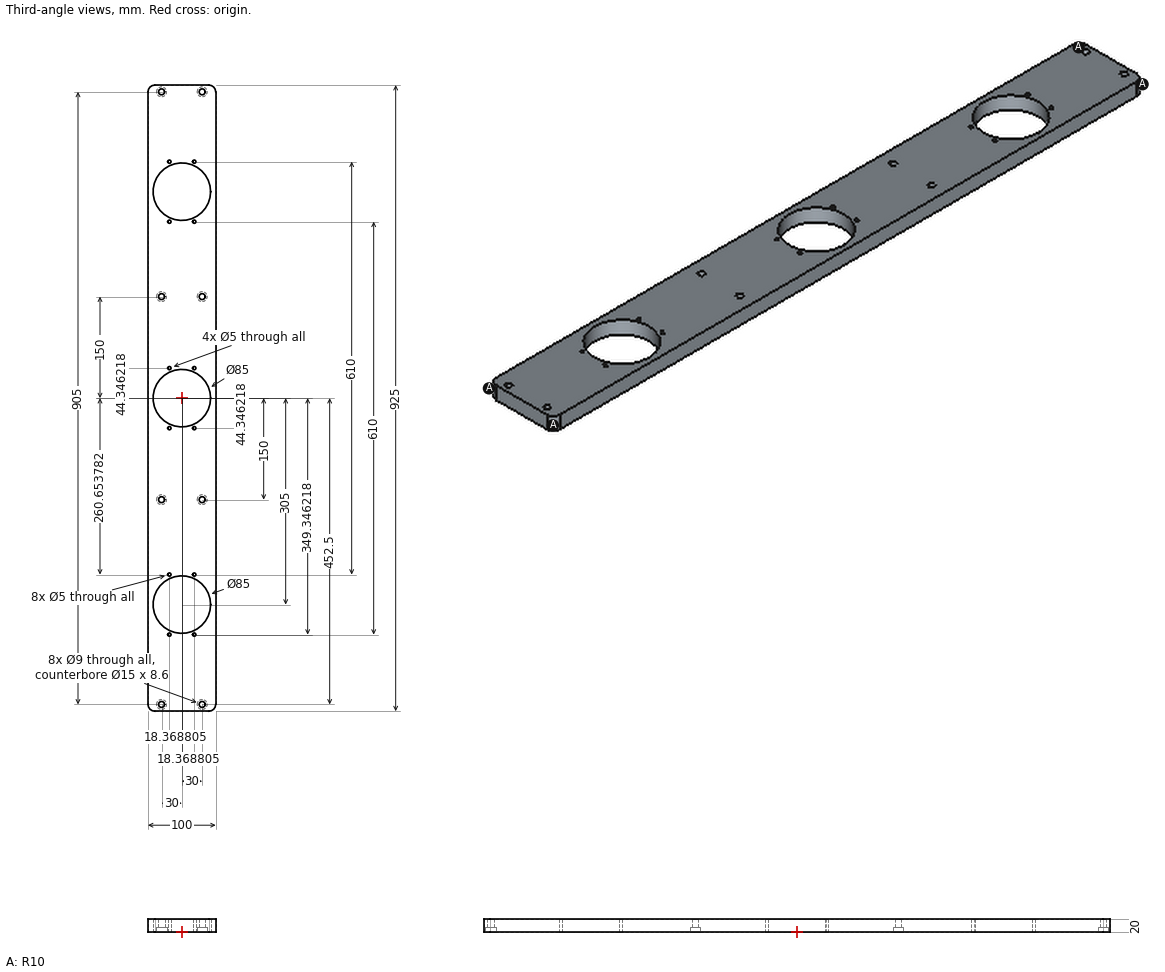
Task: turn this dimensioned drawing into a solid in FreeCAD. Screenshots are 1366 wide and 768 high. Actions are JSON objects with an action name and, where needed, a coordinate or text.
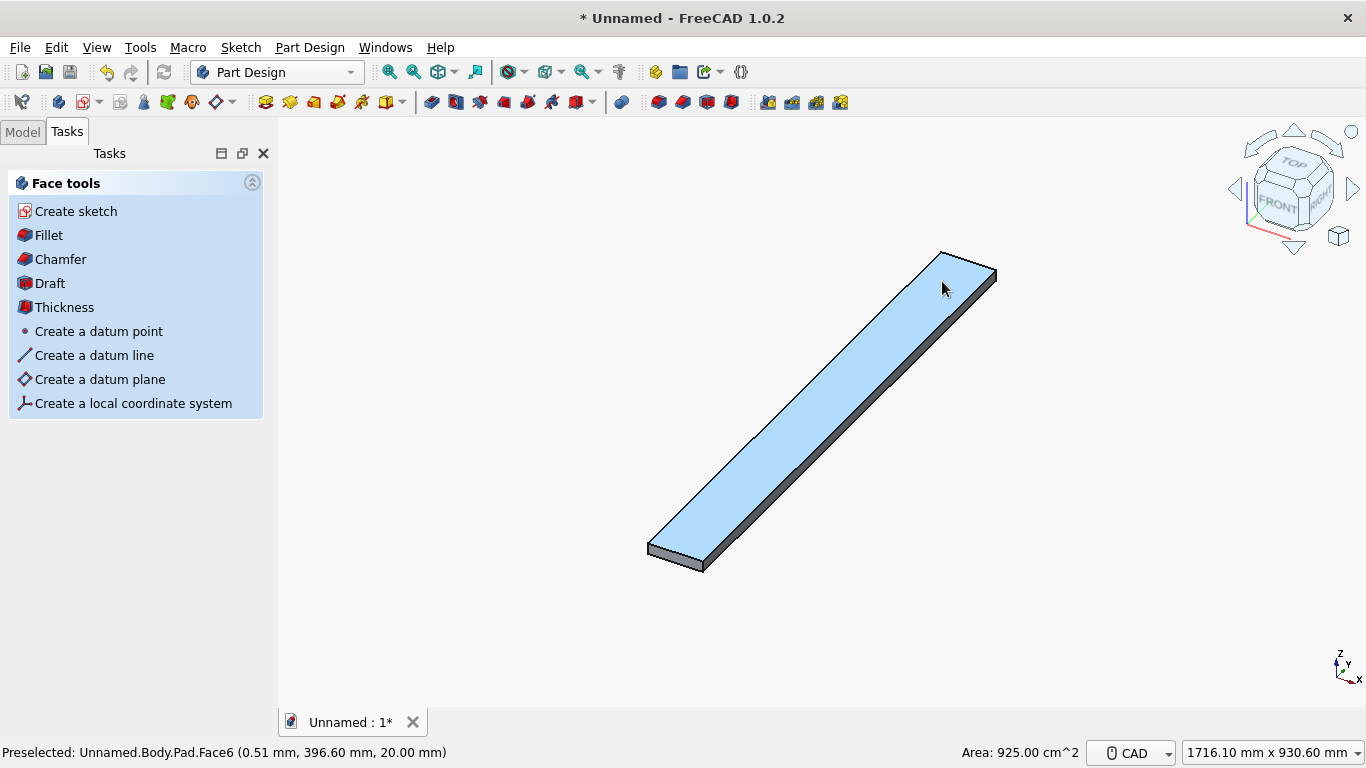
{"action": "left_click", "coordinate": [84, 102]}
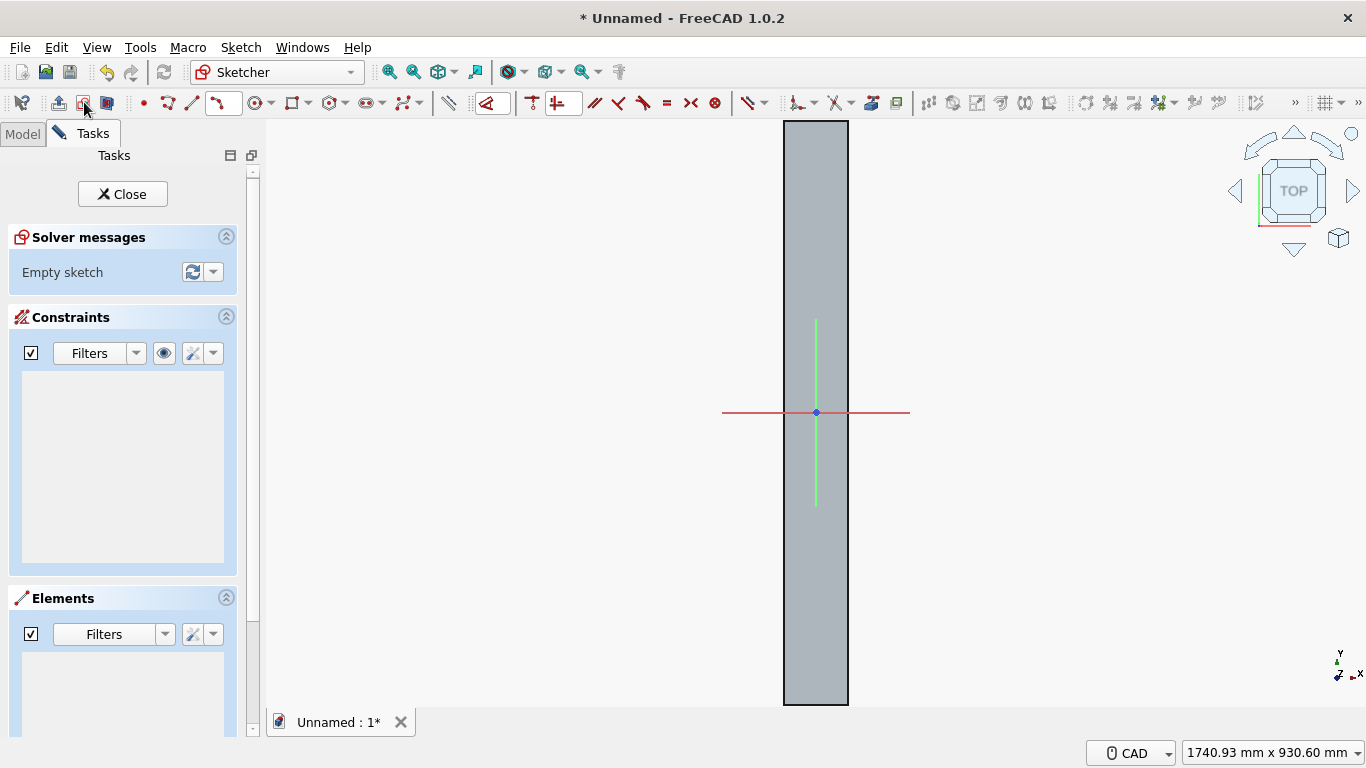
{"action": "left_click", "coordinate": [256, 104]}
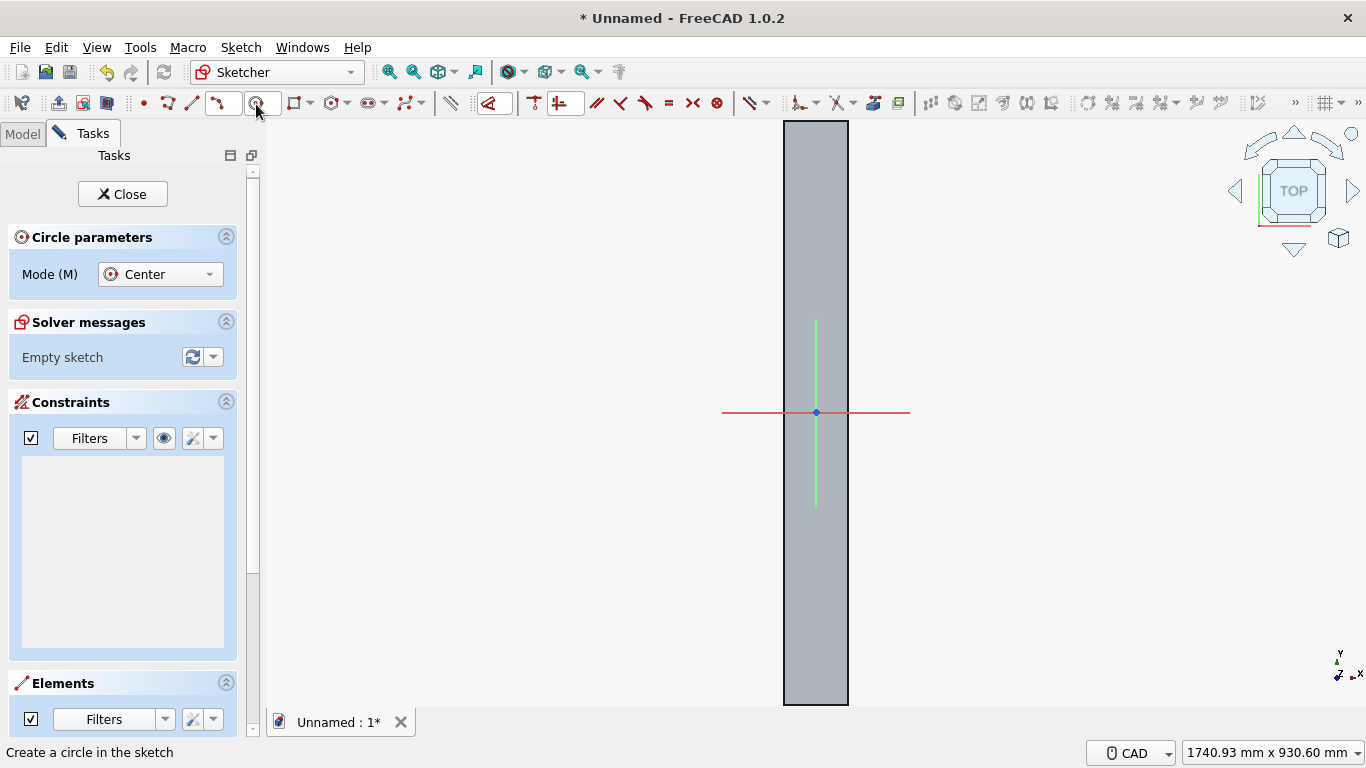
{"action": "scroll", "coordinate": [804, 578], "scroll_direction": "up", "scroll_amount": 14}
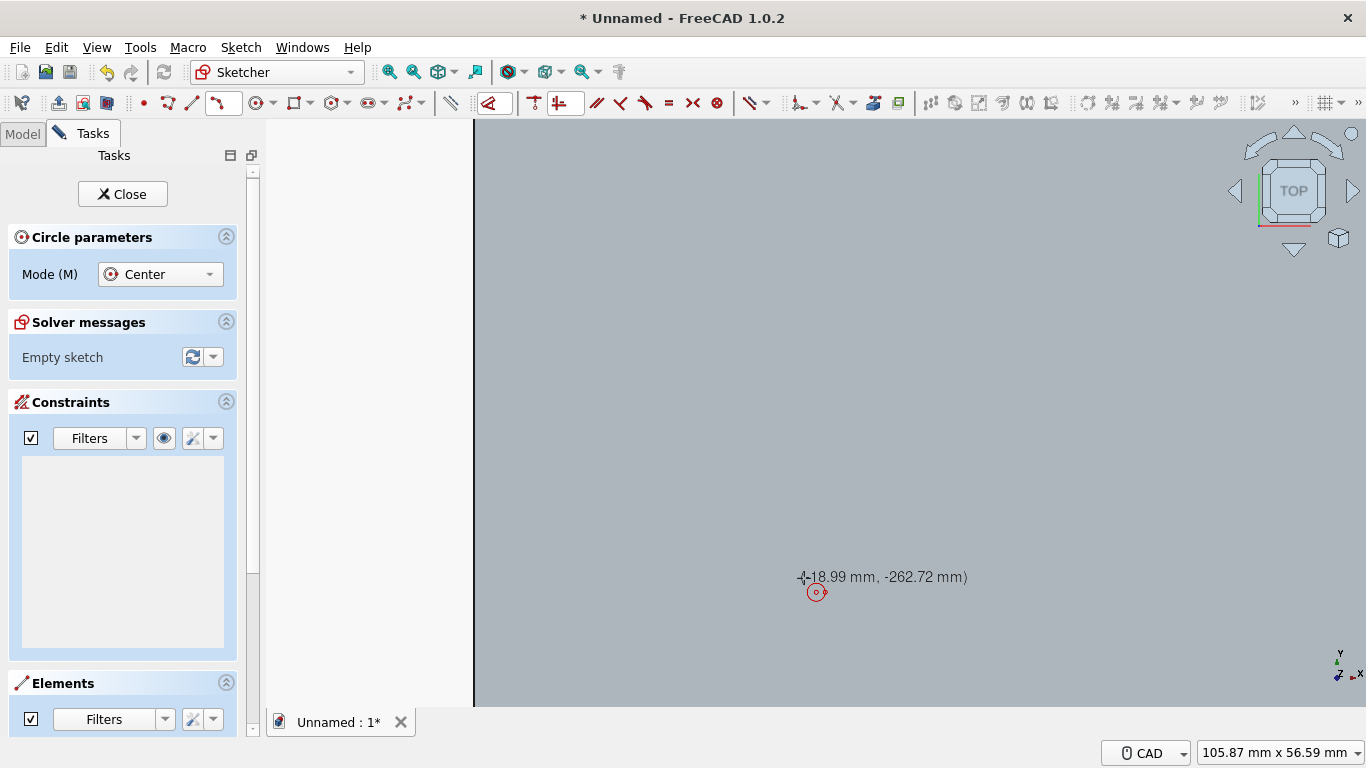
{"action": "scroll", "coordinate": [735, 547], "scroll_direction": "down", "scroll_amount": 15}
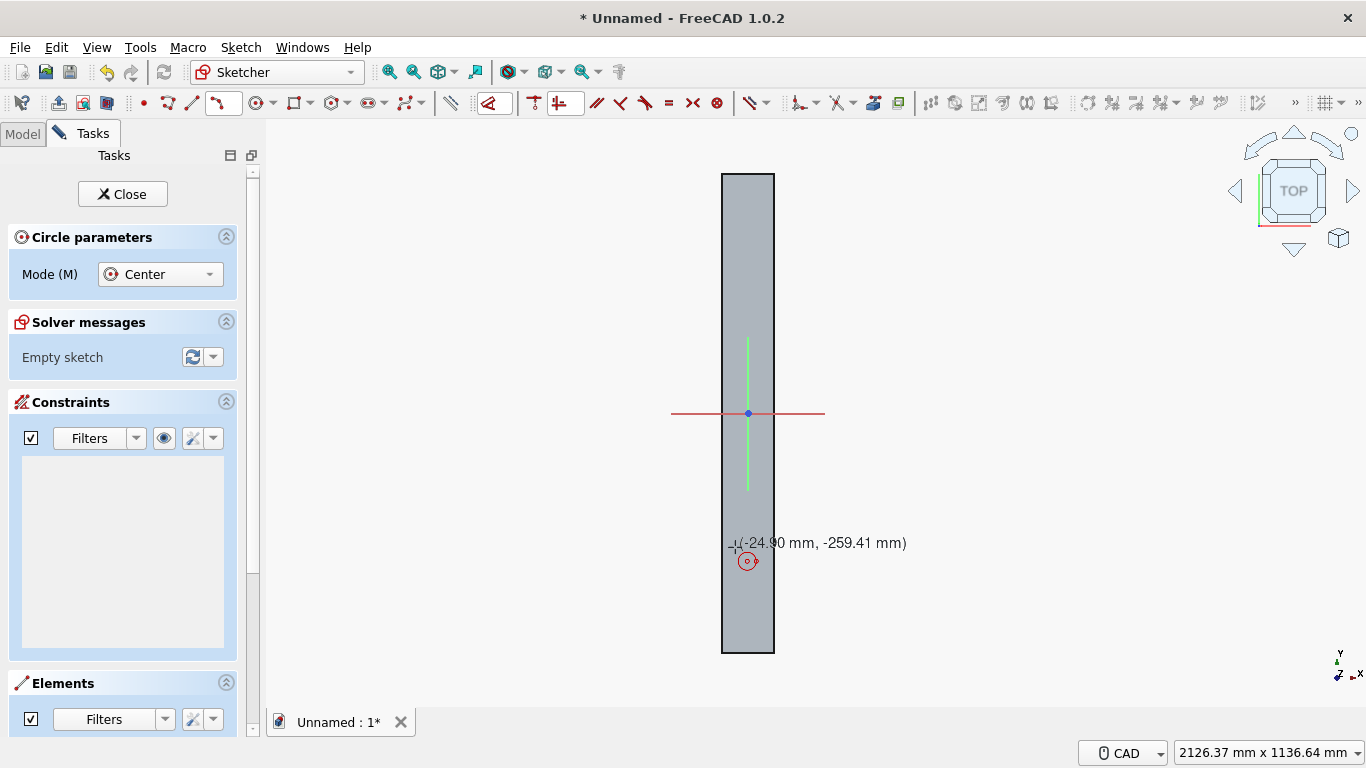
{"action": "scroll", "coordinate": [739, 548], "scroll_direction": "up", "scroll_amount": 3}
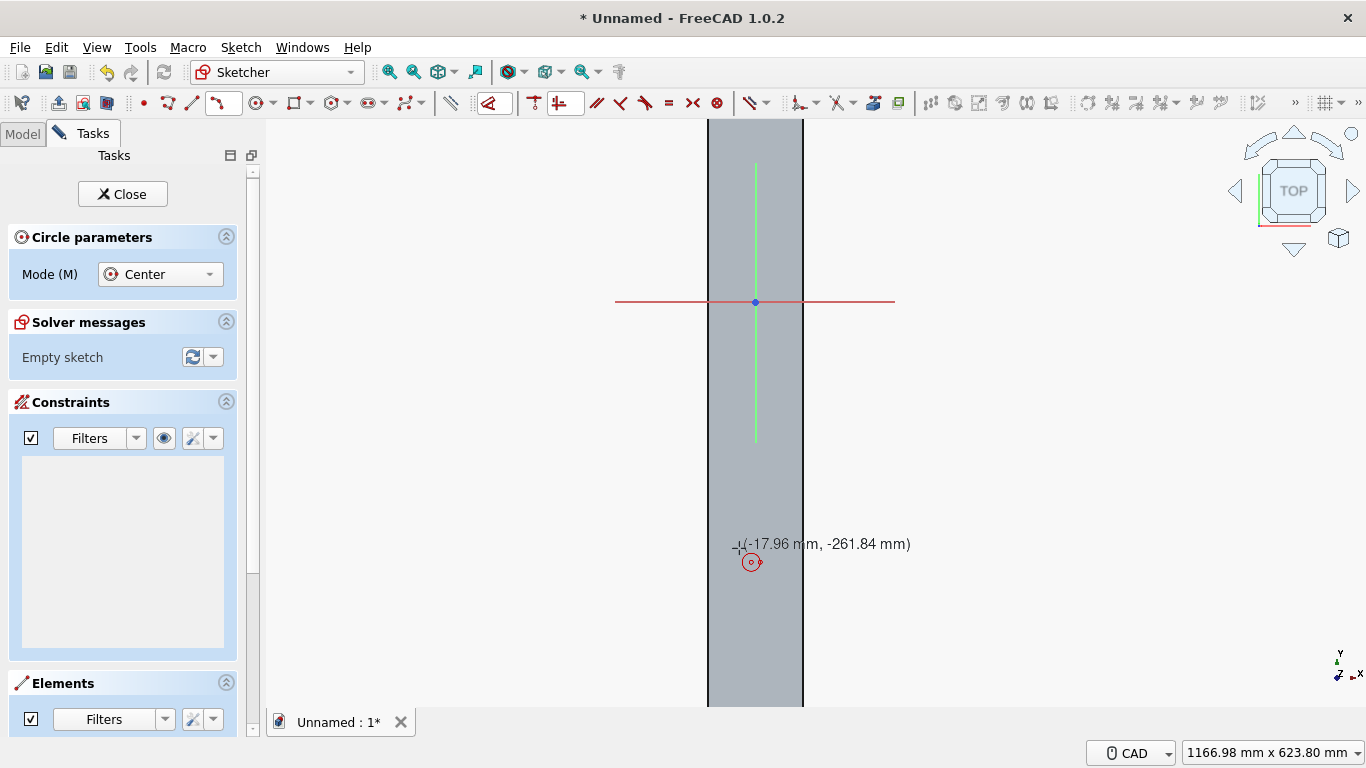
{"action": "left_click", "coordinate": [738, 548]}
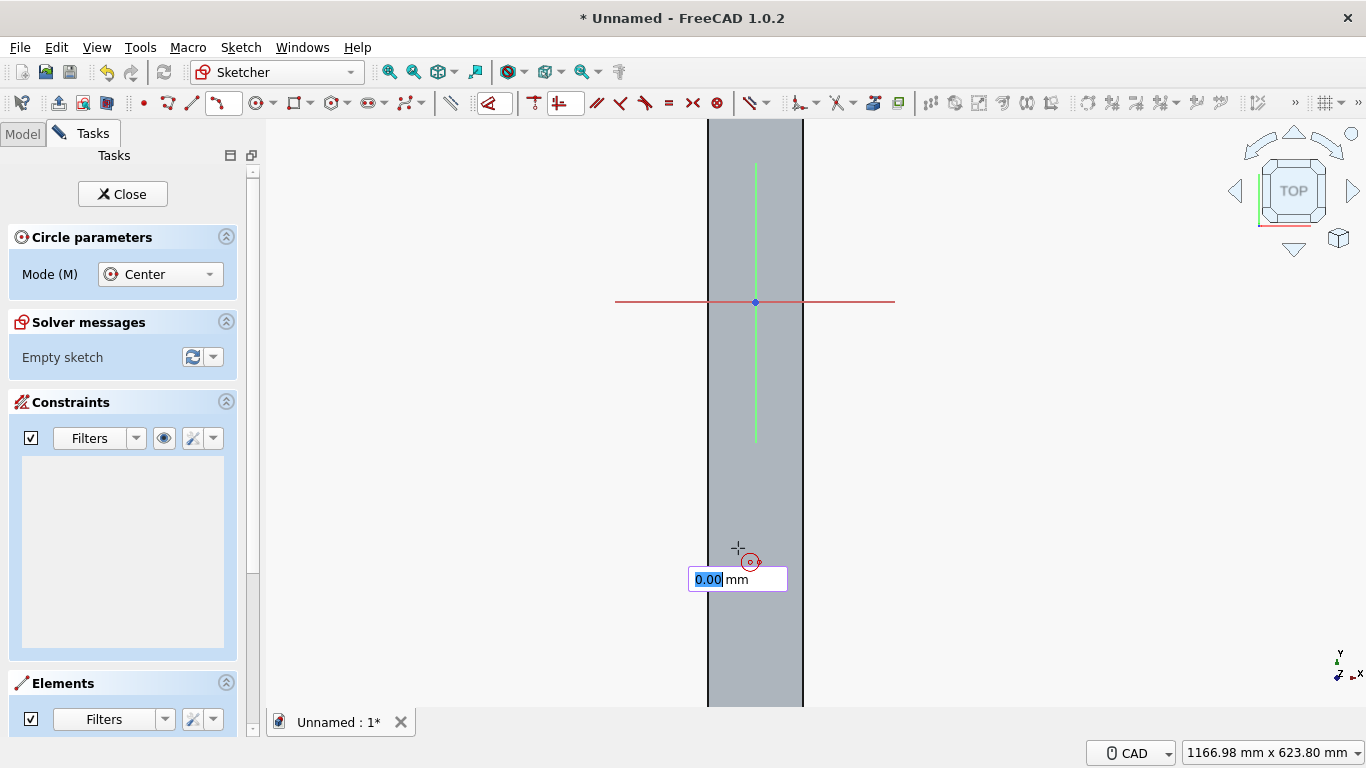
{"action": "scroll", "coordinate": [740, 546], "scroll_direction": "up", "scroll_amount": 10}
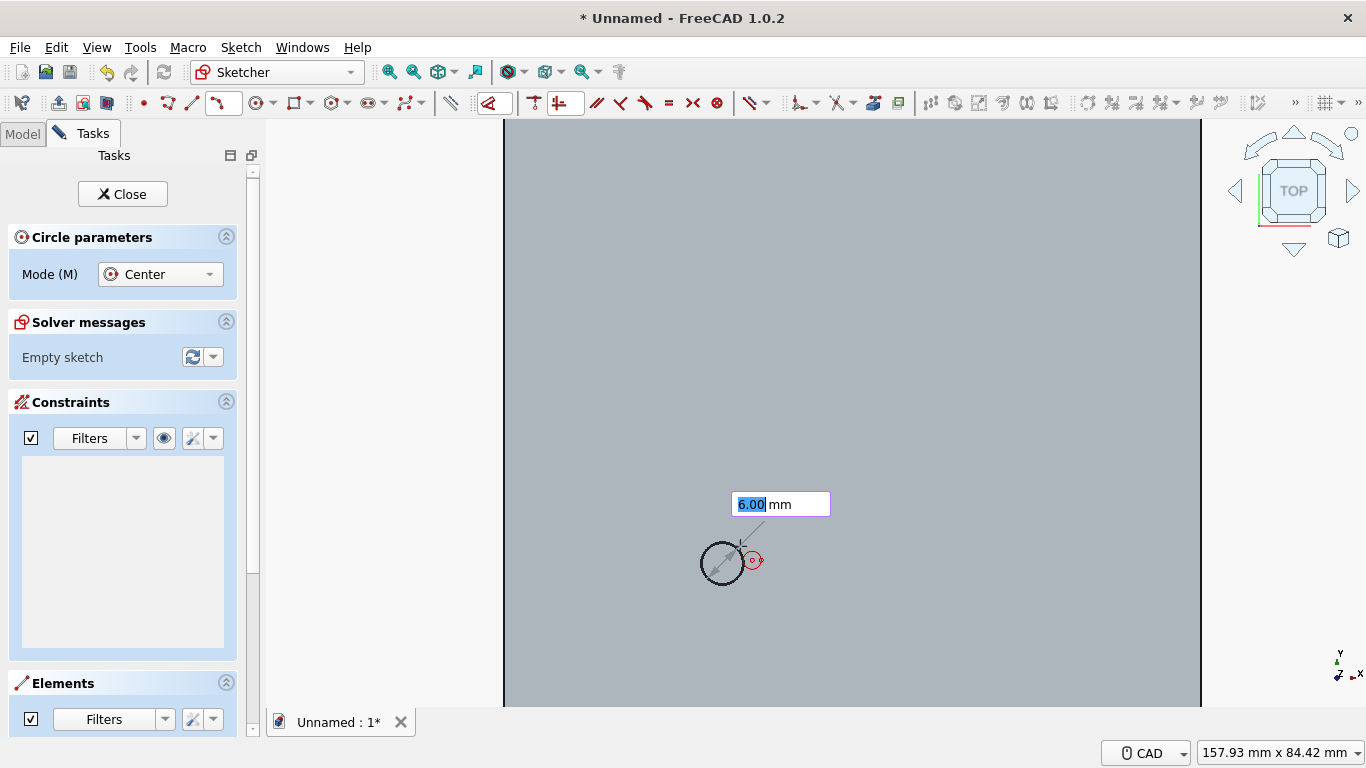
{"action": "left_click", "coordinate": [737, 545]}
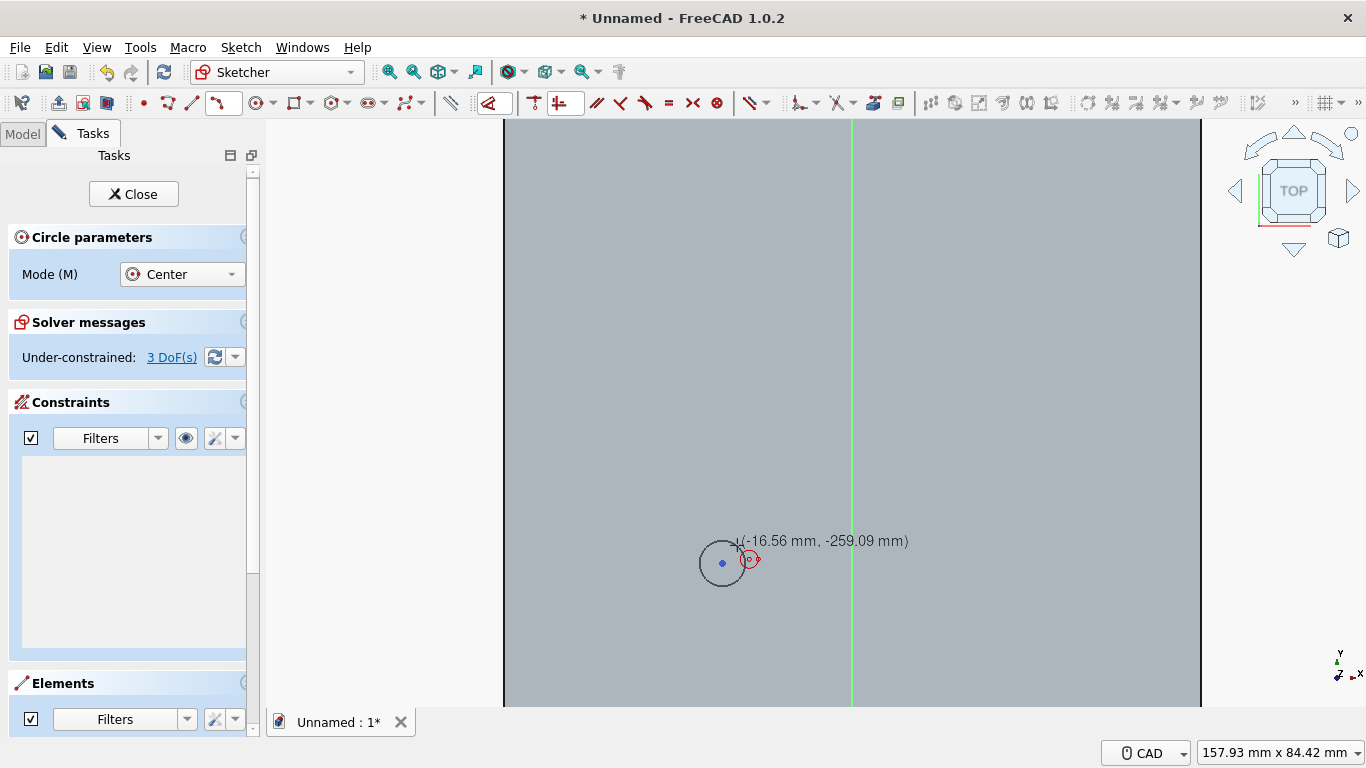
{"action": "scroll", "coordinate": [980, 557], "scroll_direction": "up", "scroll_amount": 2}